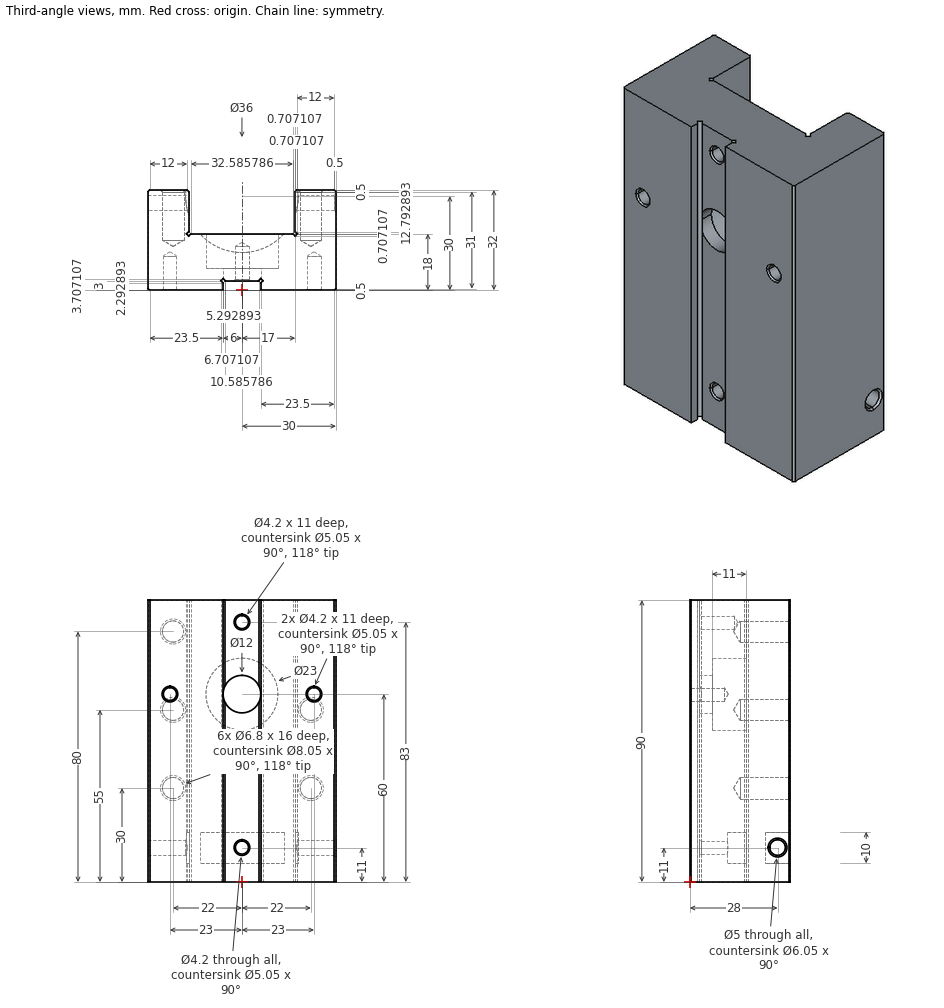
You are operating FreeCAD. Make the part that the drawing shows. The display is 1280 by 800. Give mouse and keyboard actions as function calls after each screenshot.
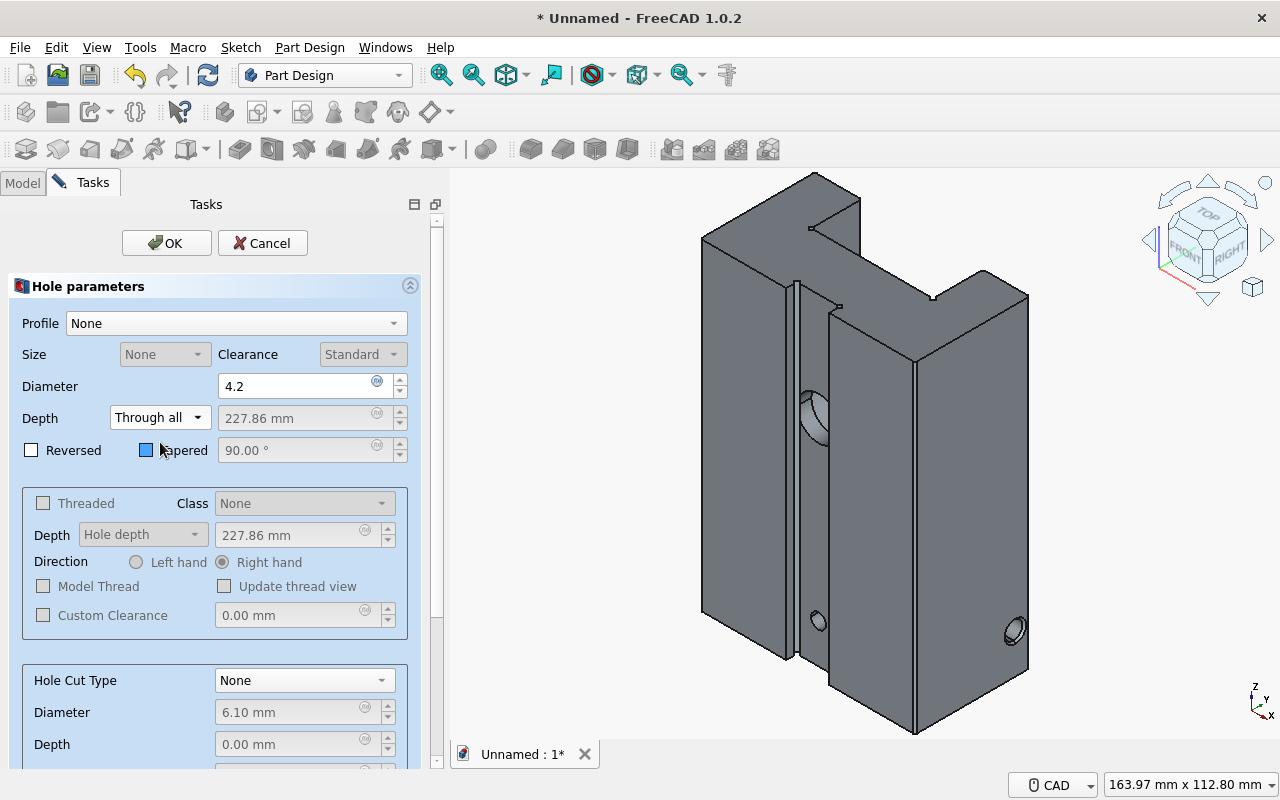
click(306, 680)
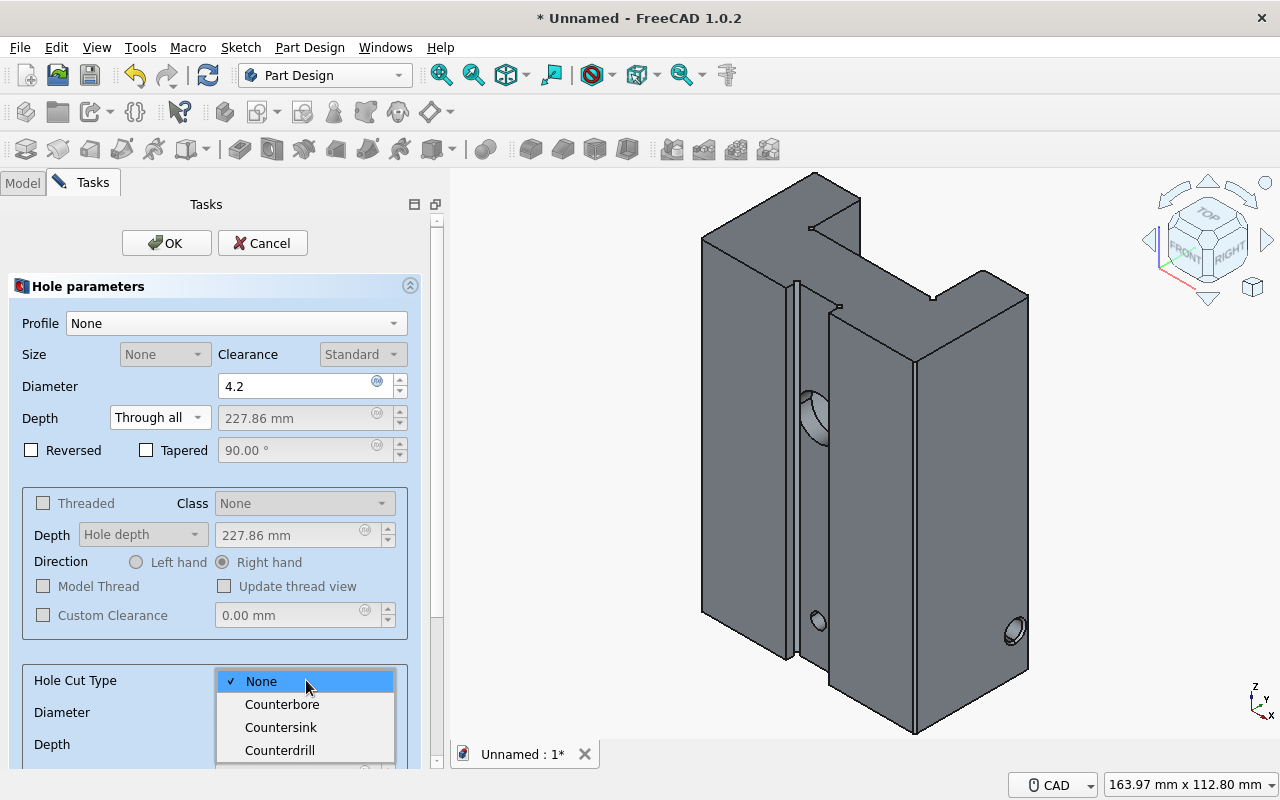
click(304, 728)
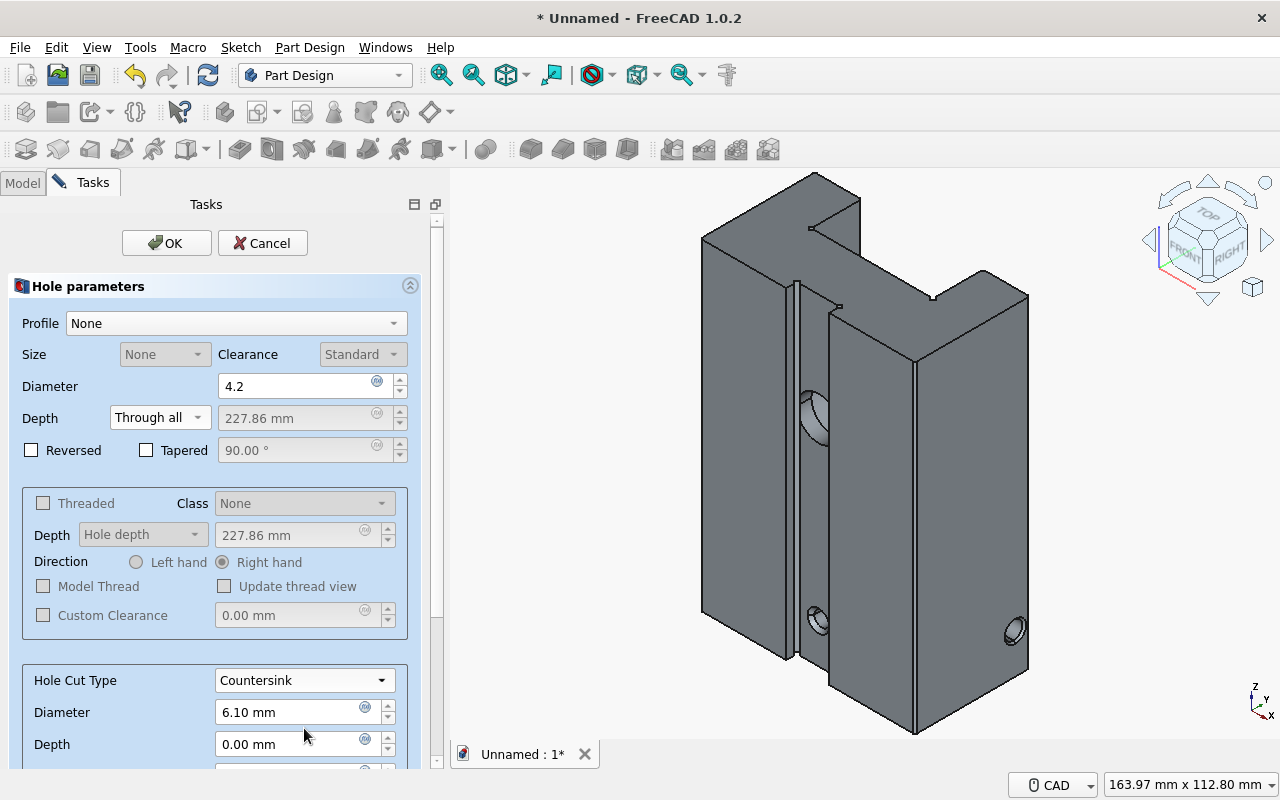
triple_click(298, 712)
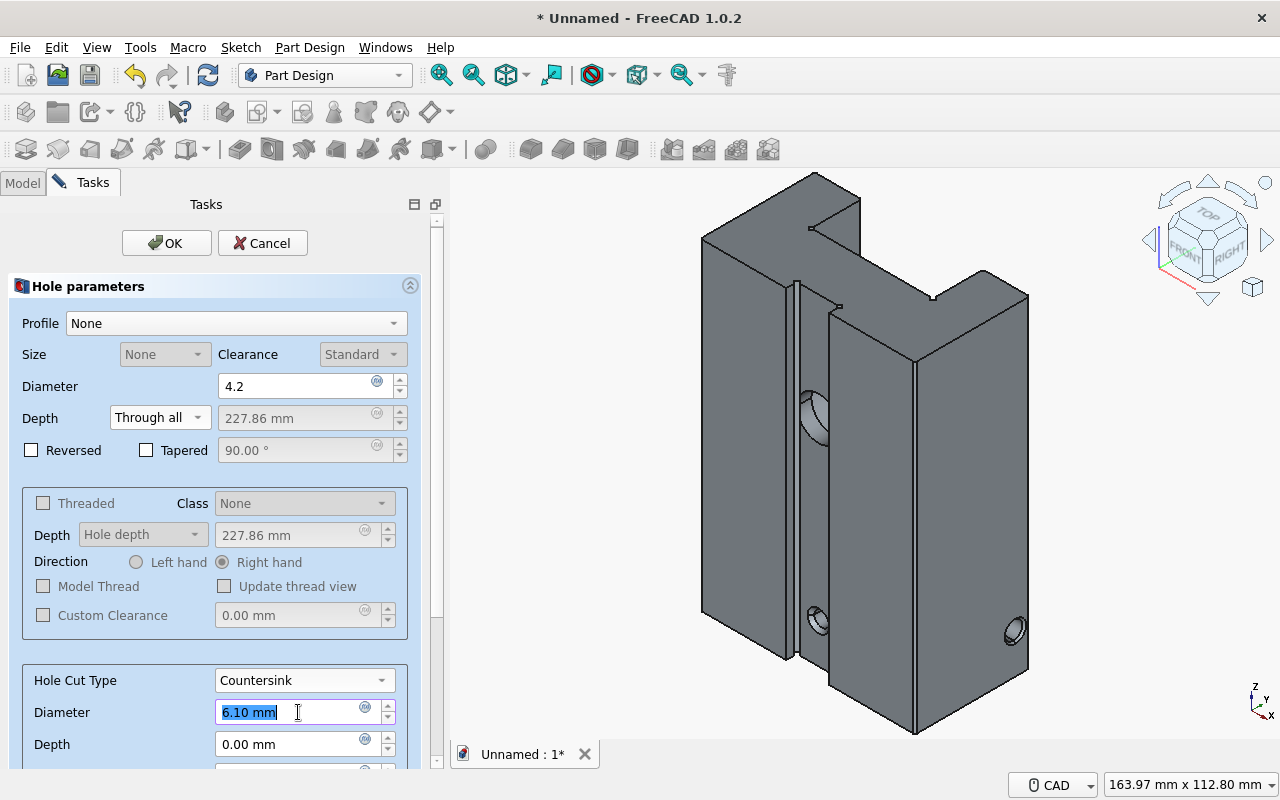
text(5.05)
key(Tab)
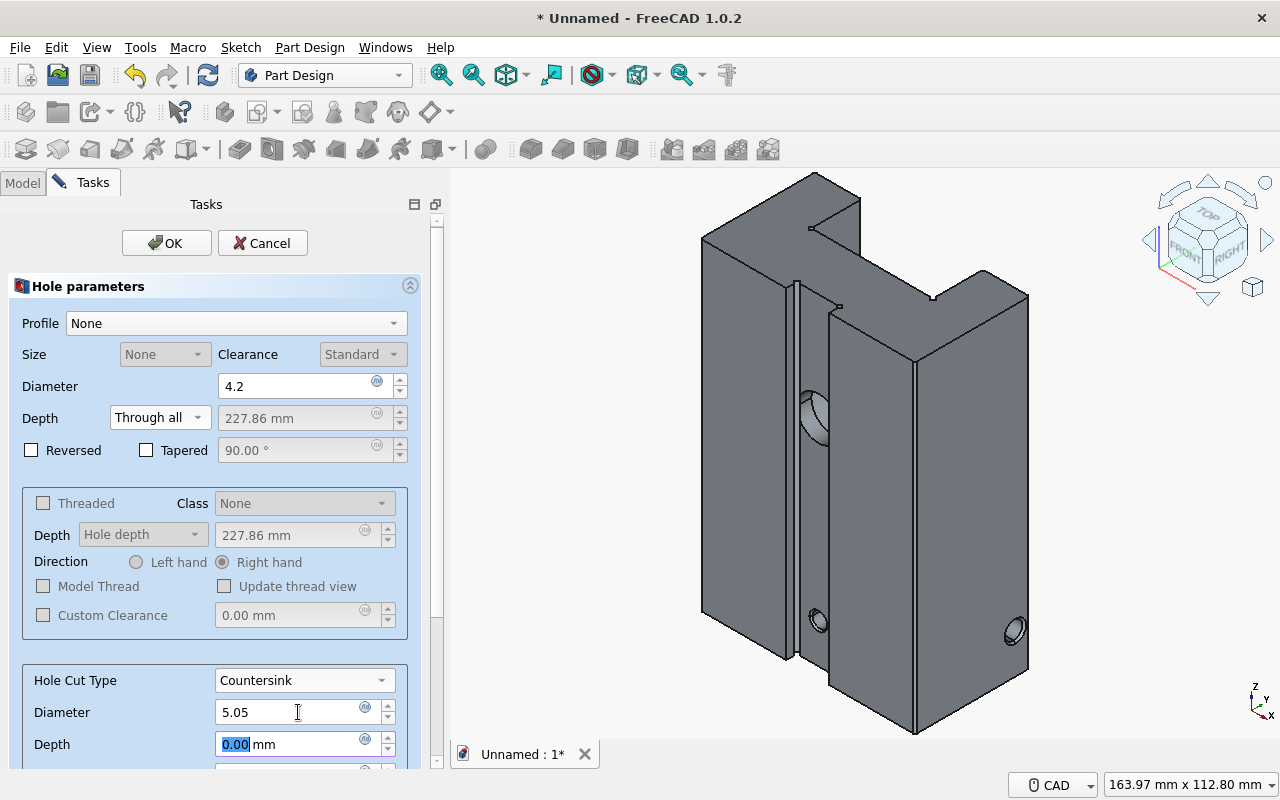
click(167, 243)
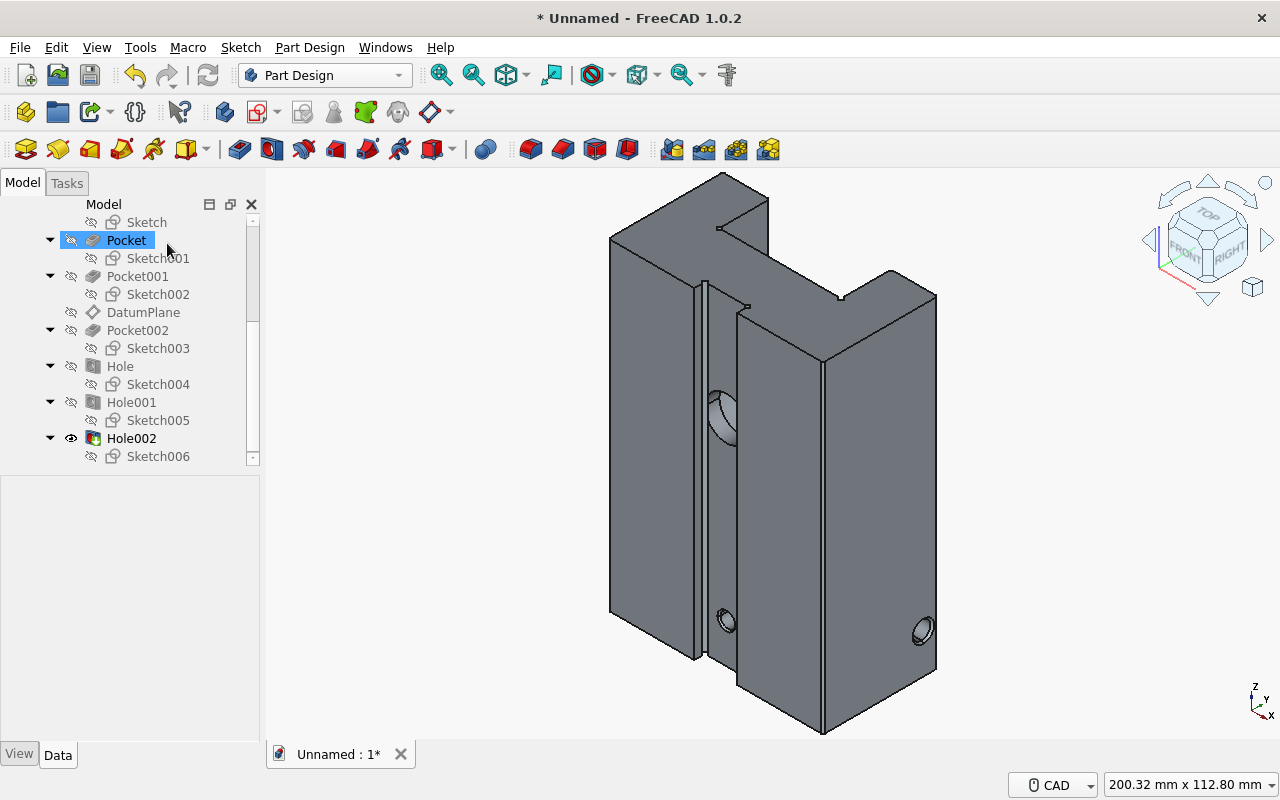
click(726, 480)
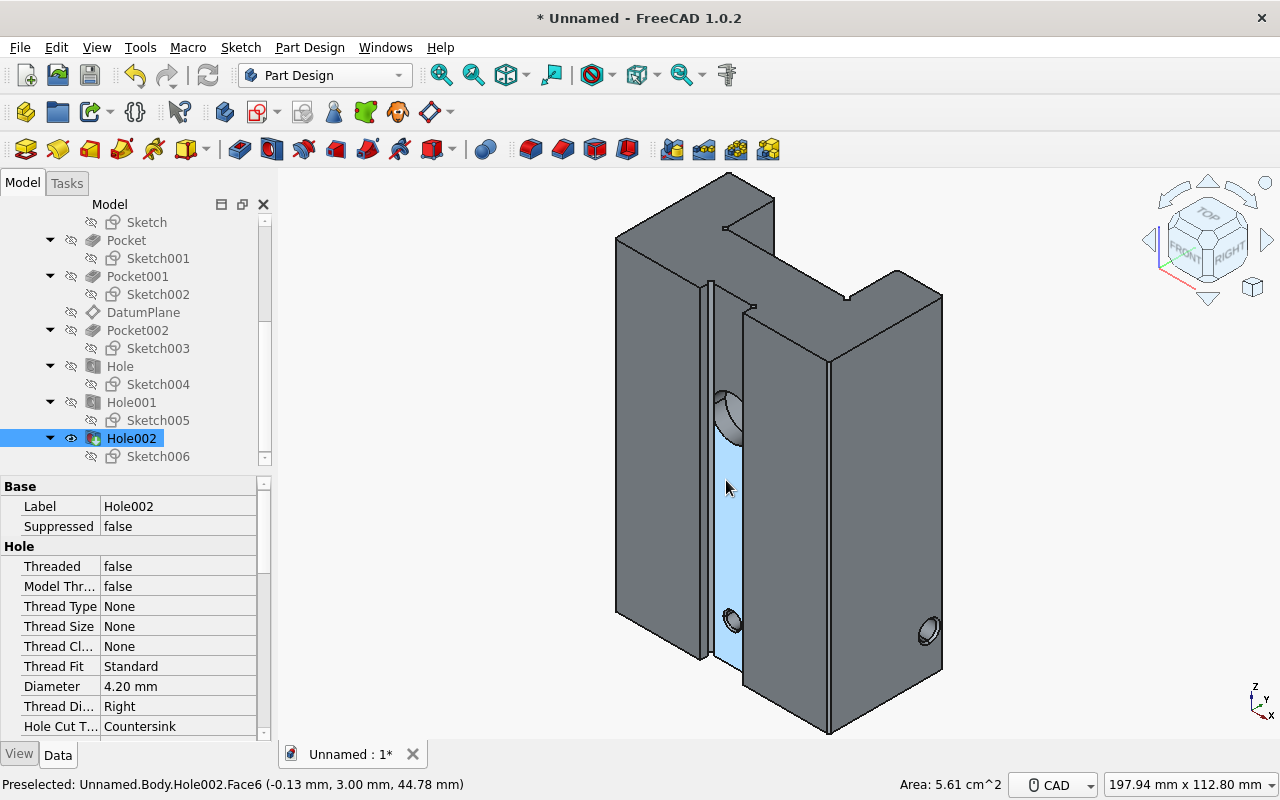
click(258, 112)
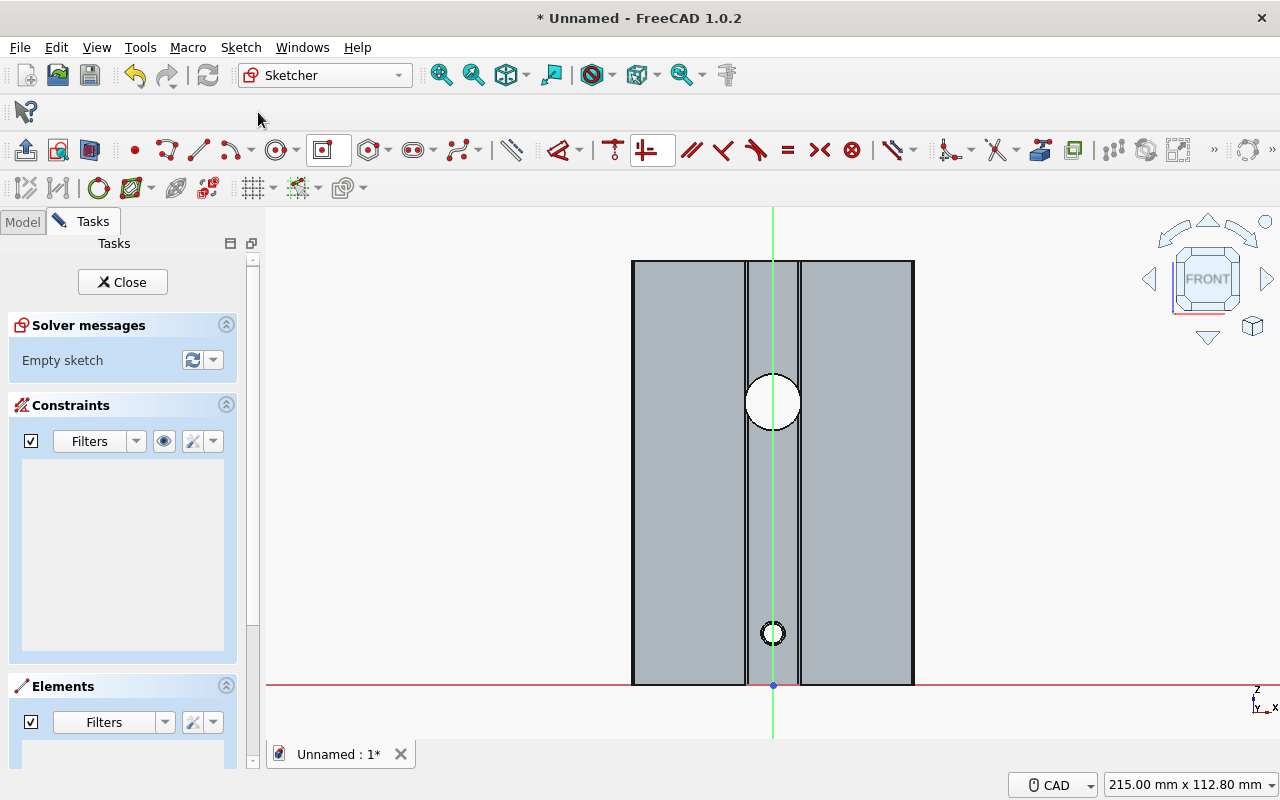
click(90, 150)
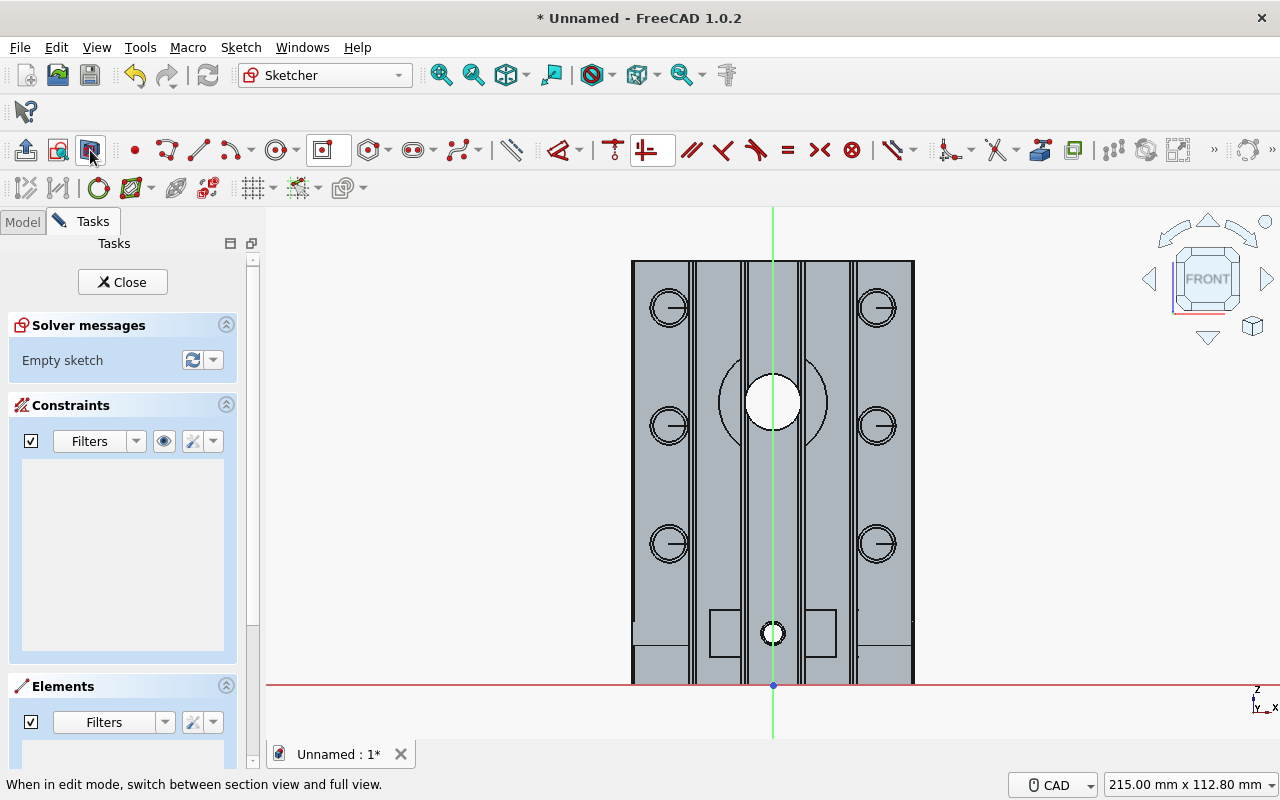
scroll(777, 282, up, 14)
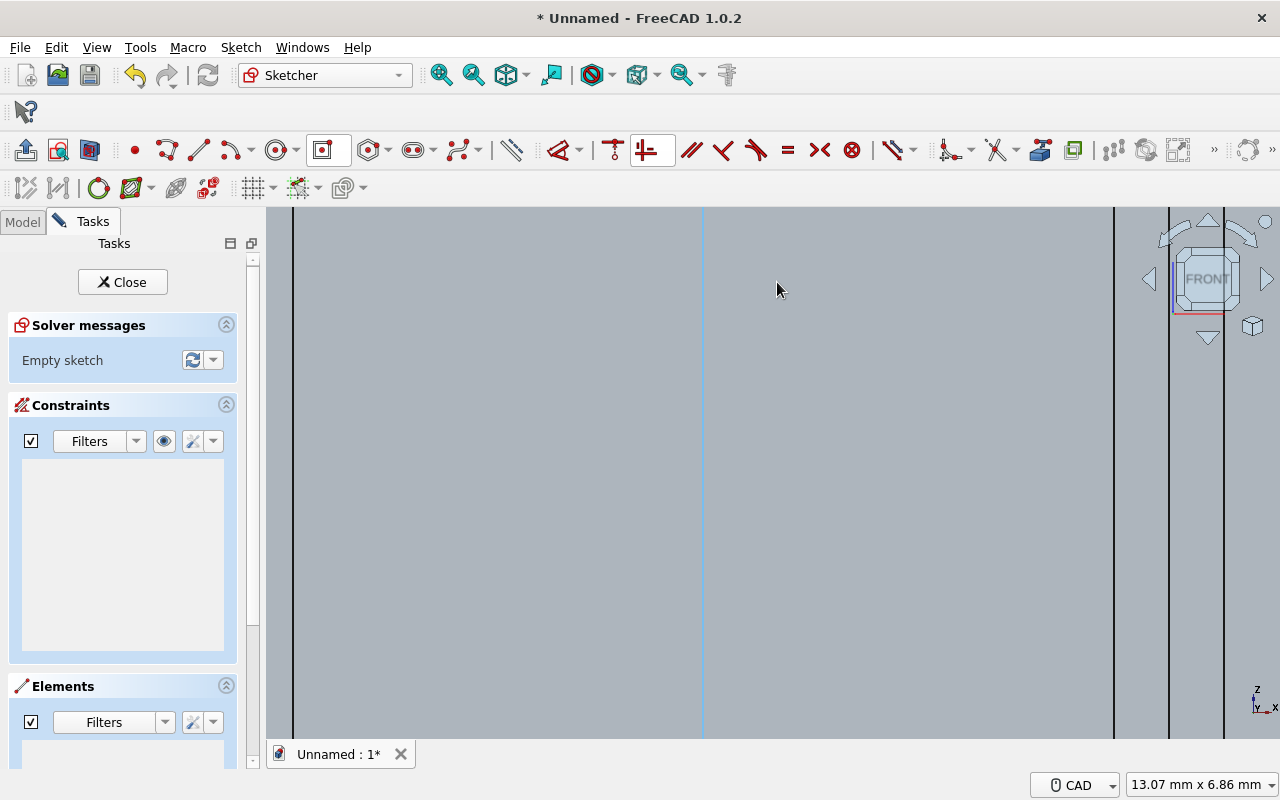
click(276, 150)